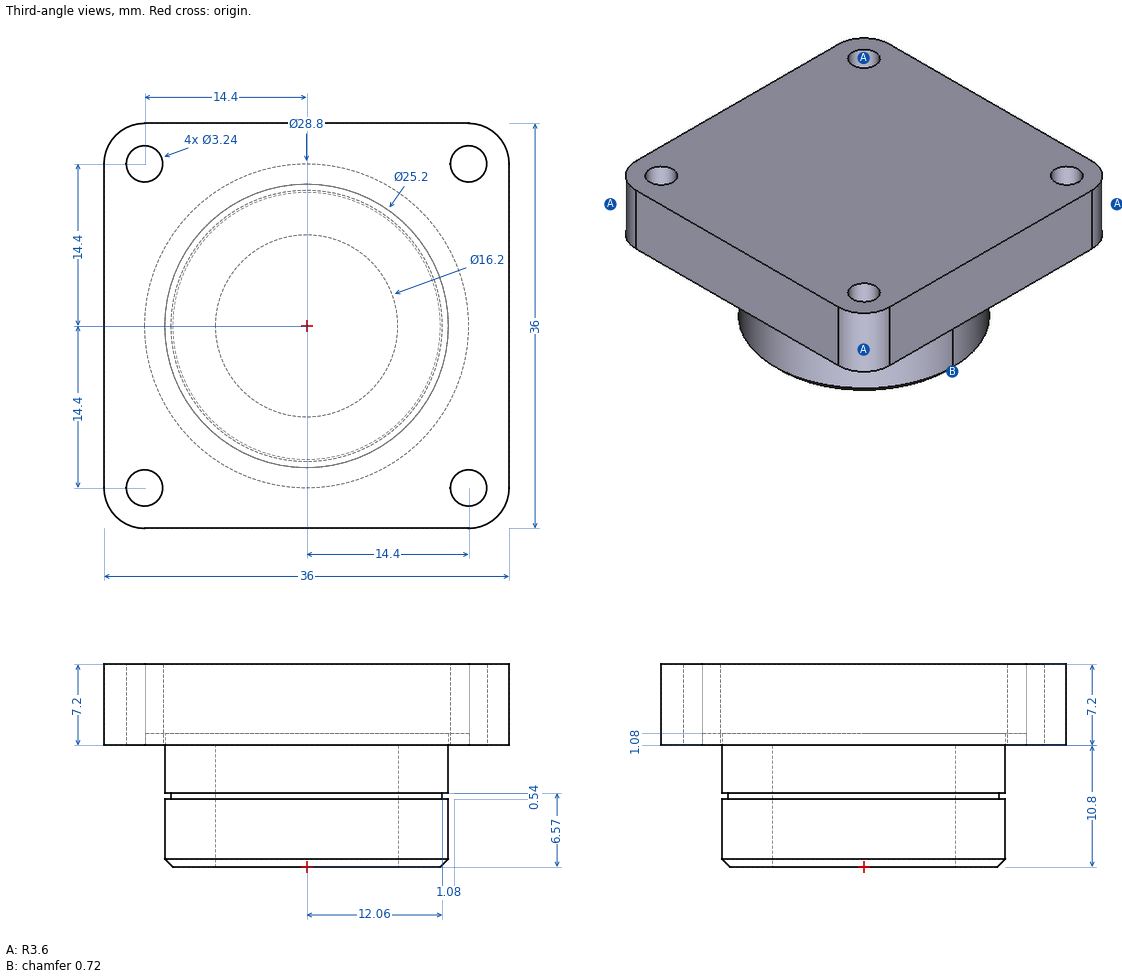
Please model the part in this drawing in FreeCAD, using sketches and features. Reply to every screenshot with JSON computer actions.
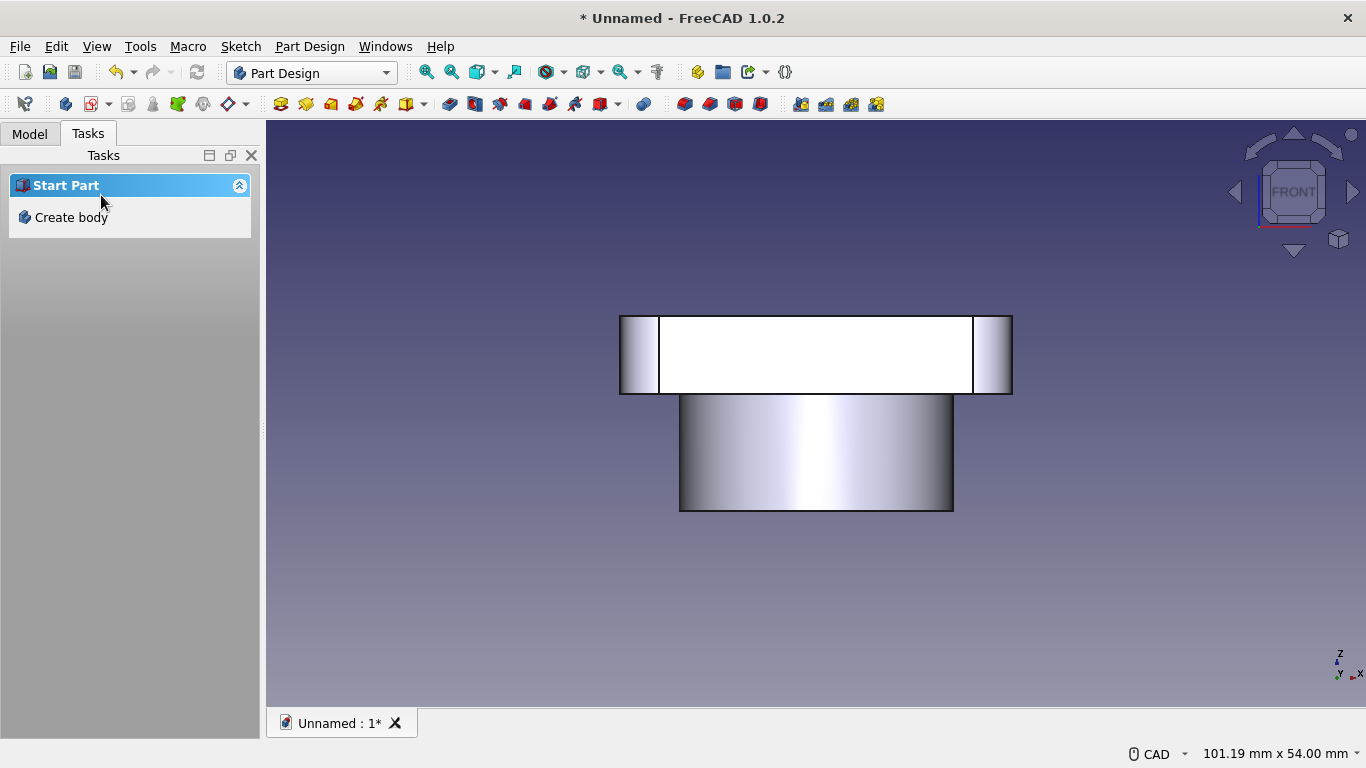
{"action": "left_click", "coordinate": [427, 72]}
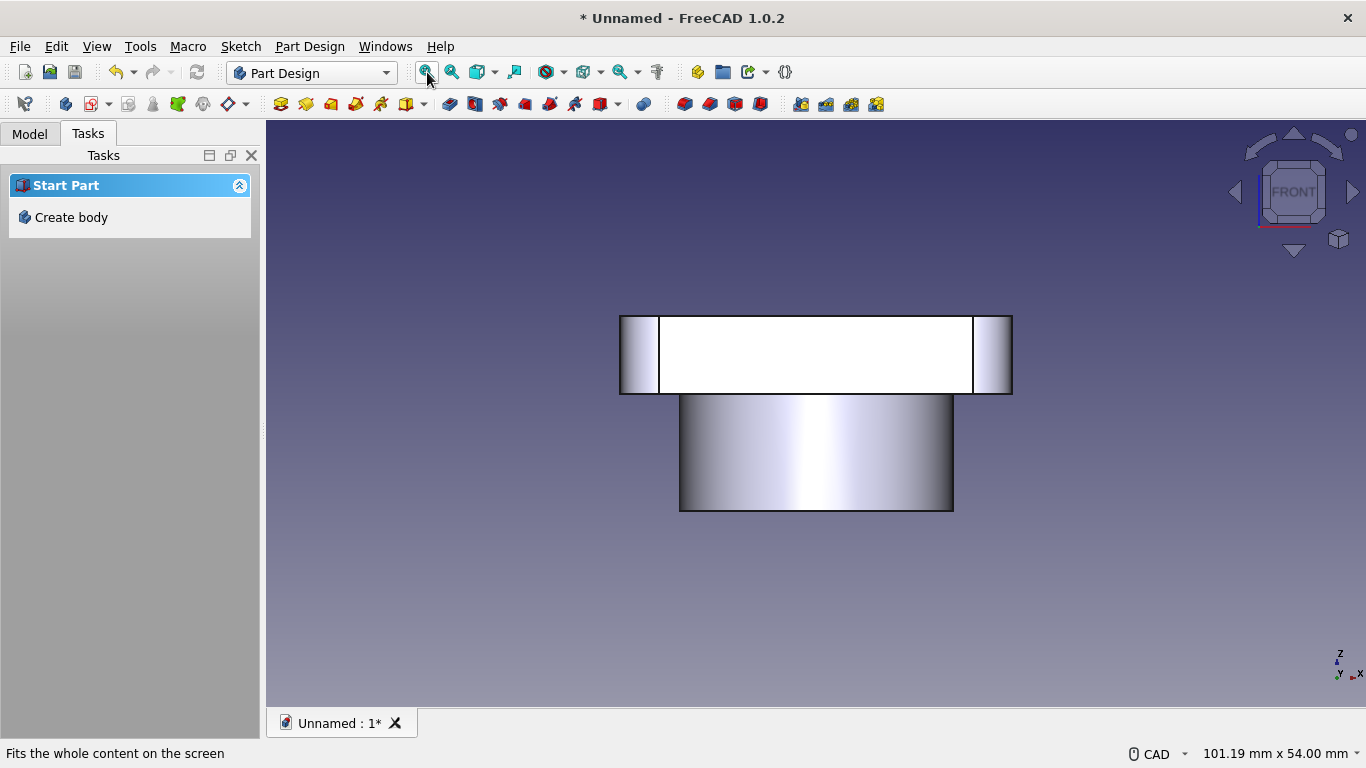
{"action": "key", "text": "3"}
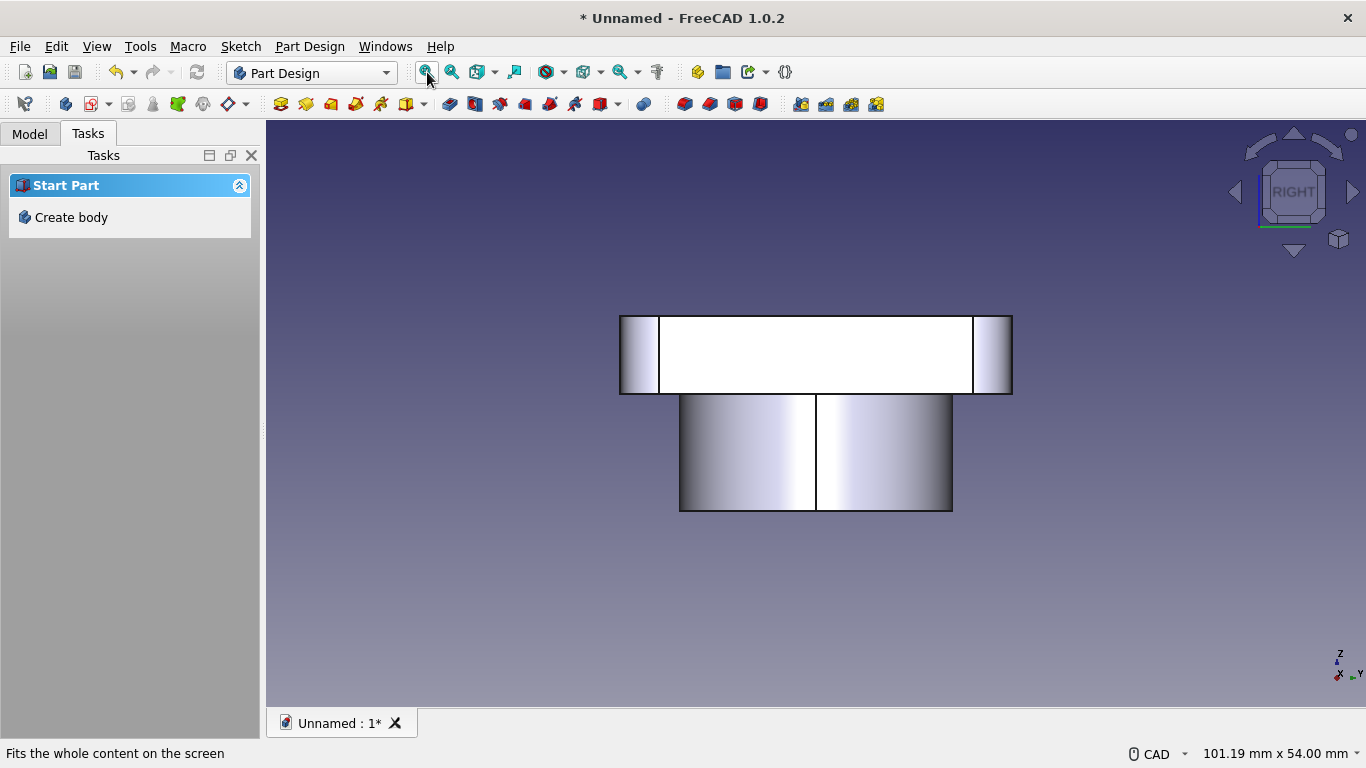
{"action": "left_click", "coordinate": [427, 72]}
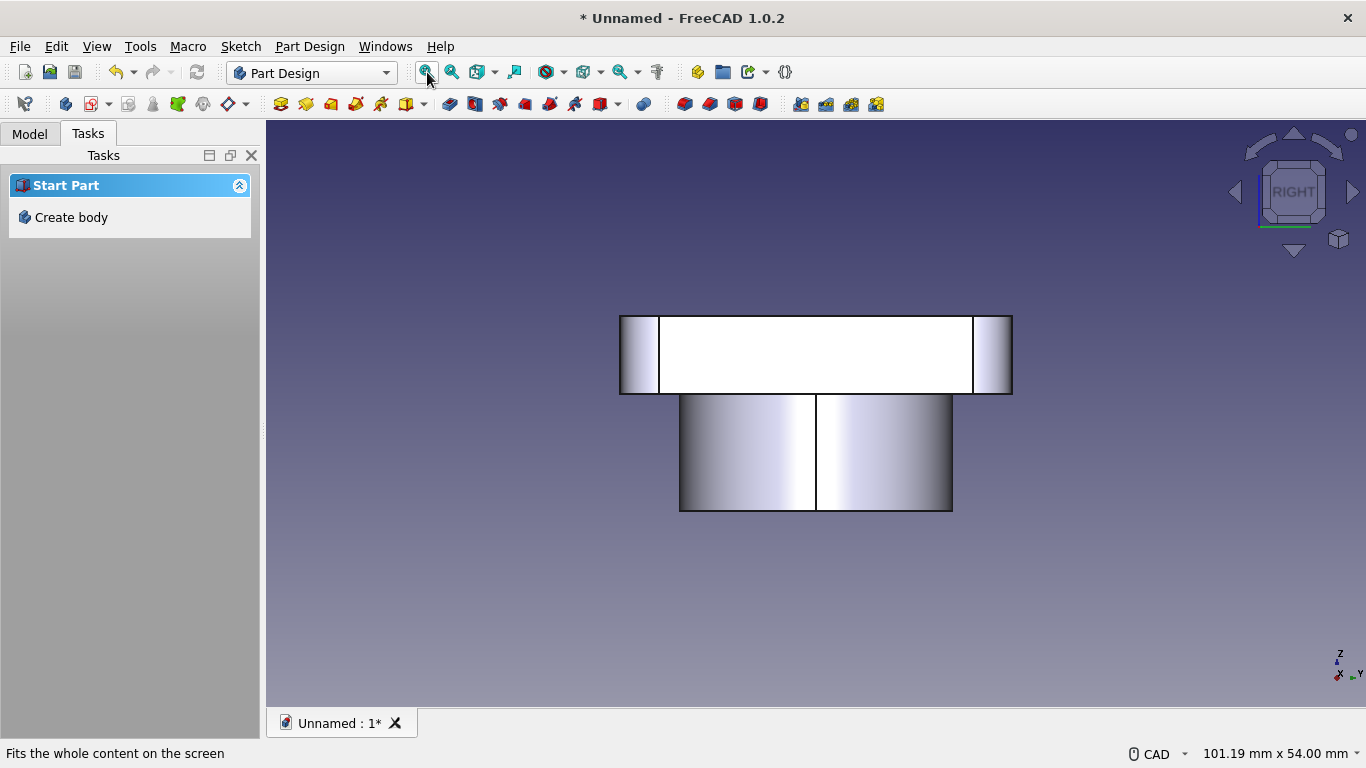
{"action": "key", "text": "5"}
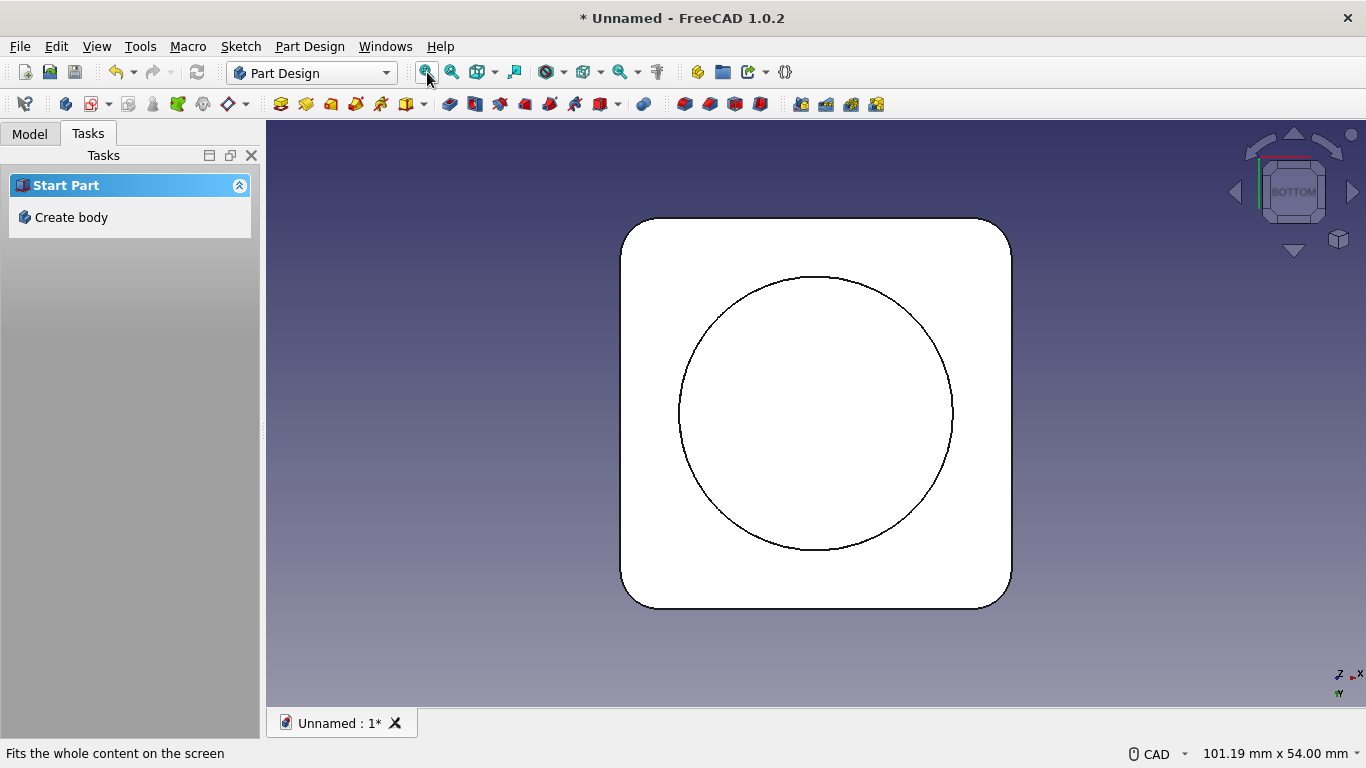
{"action": "left_click", "coordinate": [679, 412]}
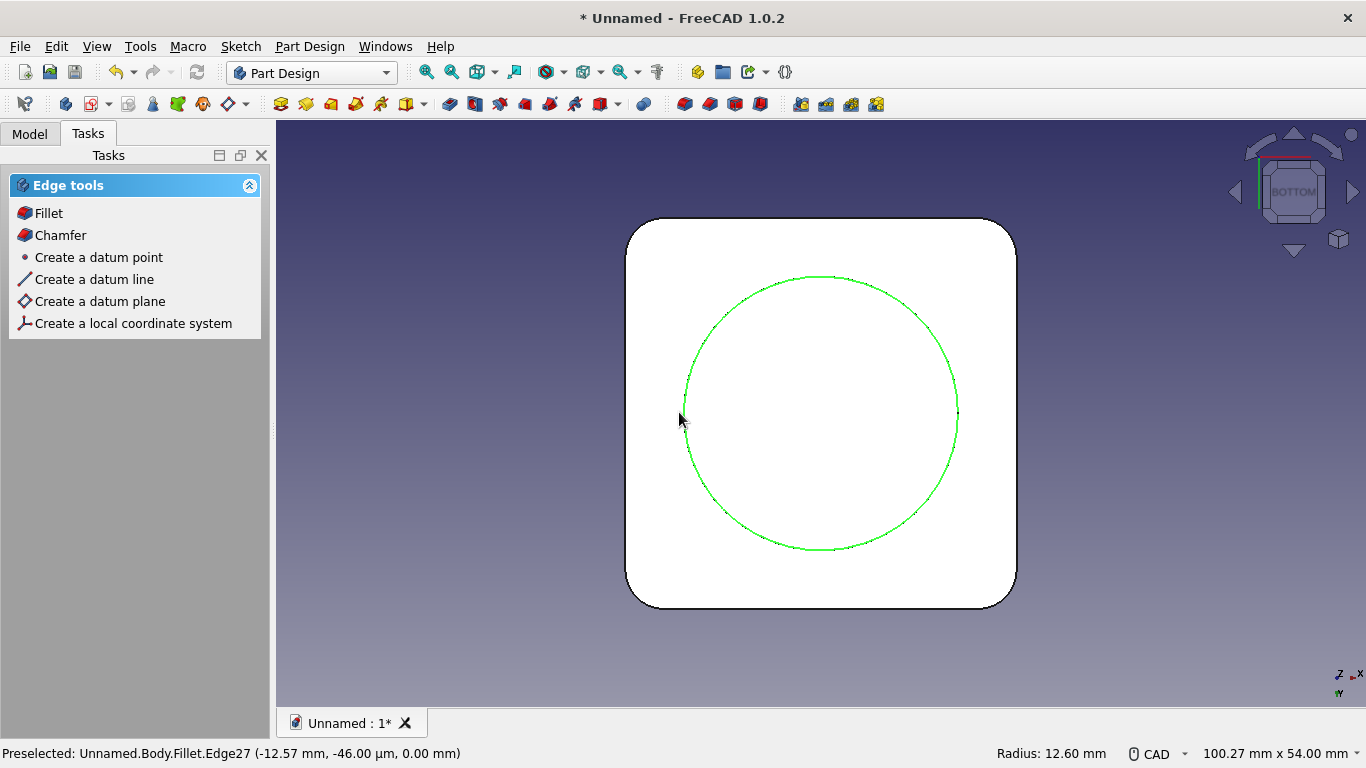
{"action": "left_click", "coordinate": [710, 104]}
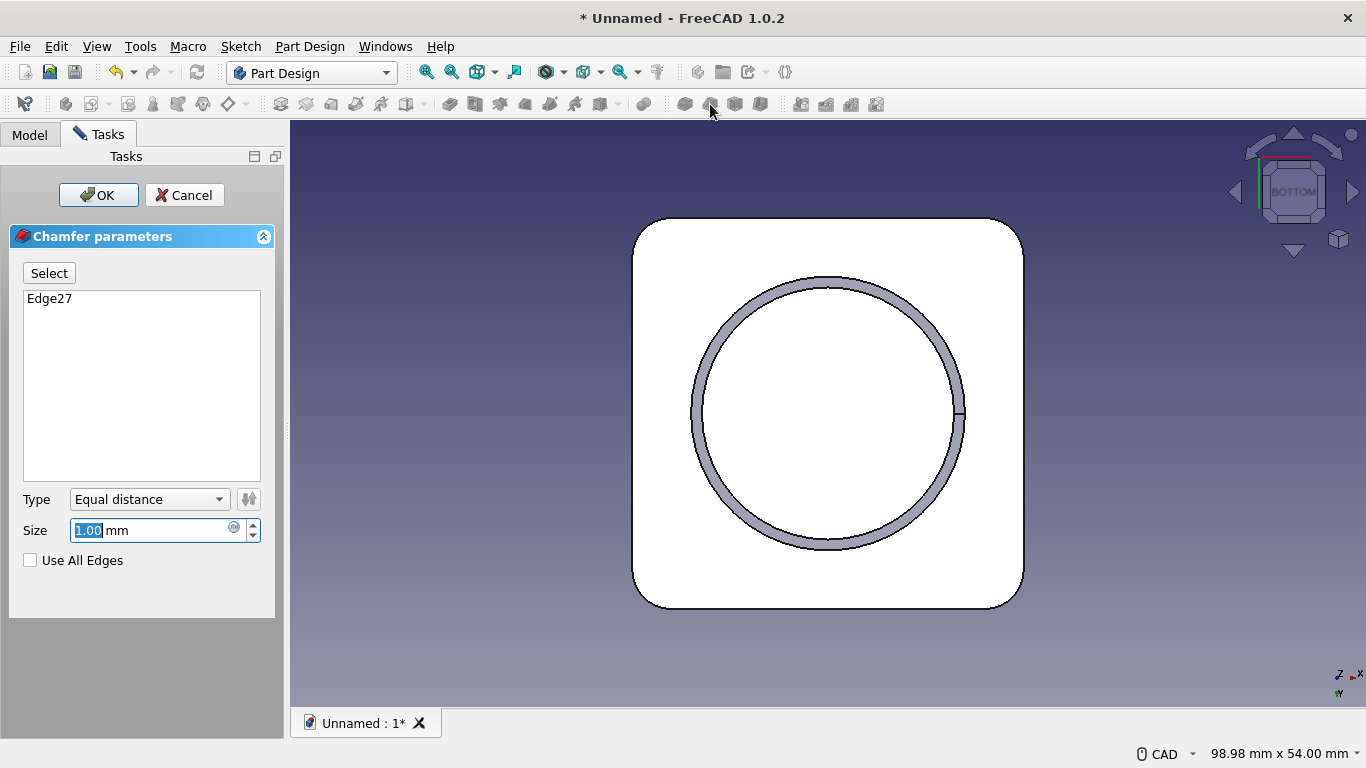
{"action": "type", "text": "0.72"}
{"action": "key", "text": "Tab"}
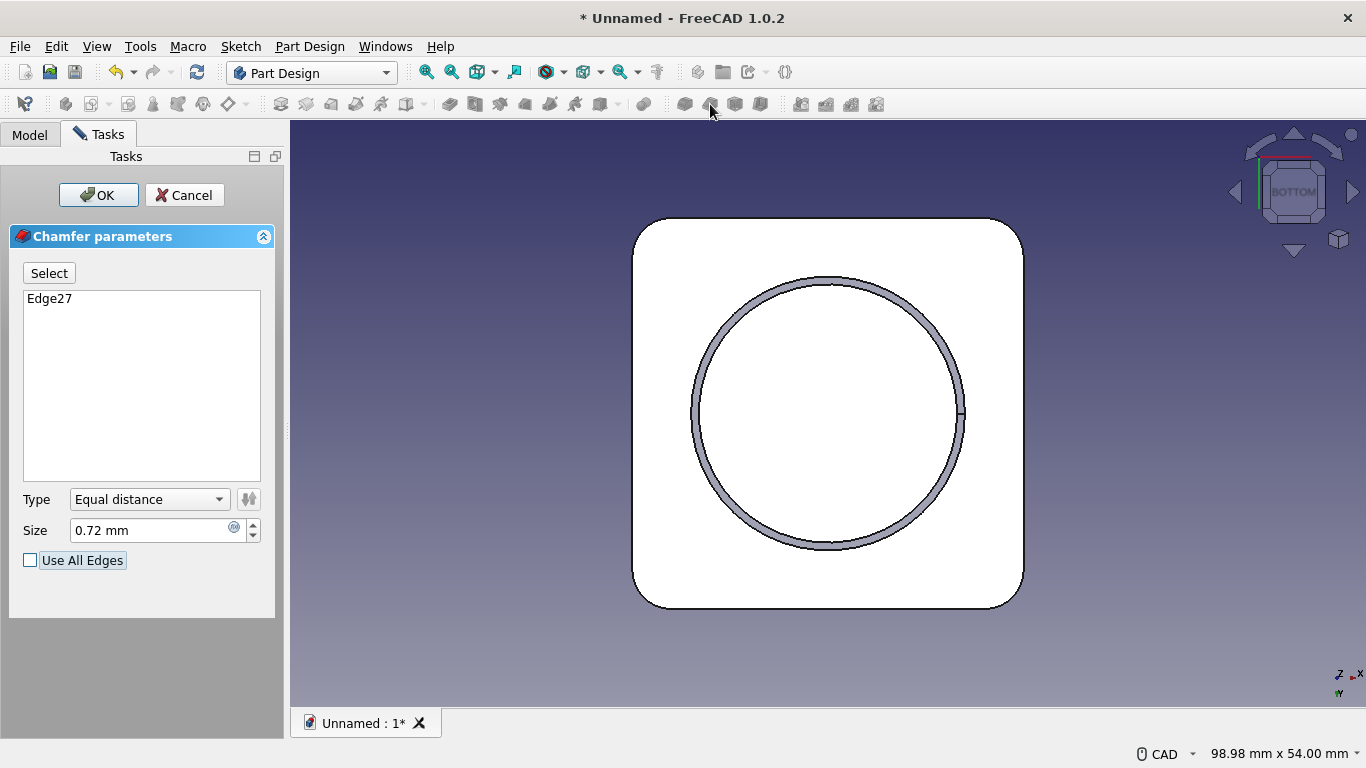
{"action": "left_click", "coordinate": [99, 195]}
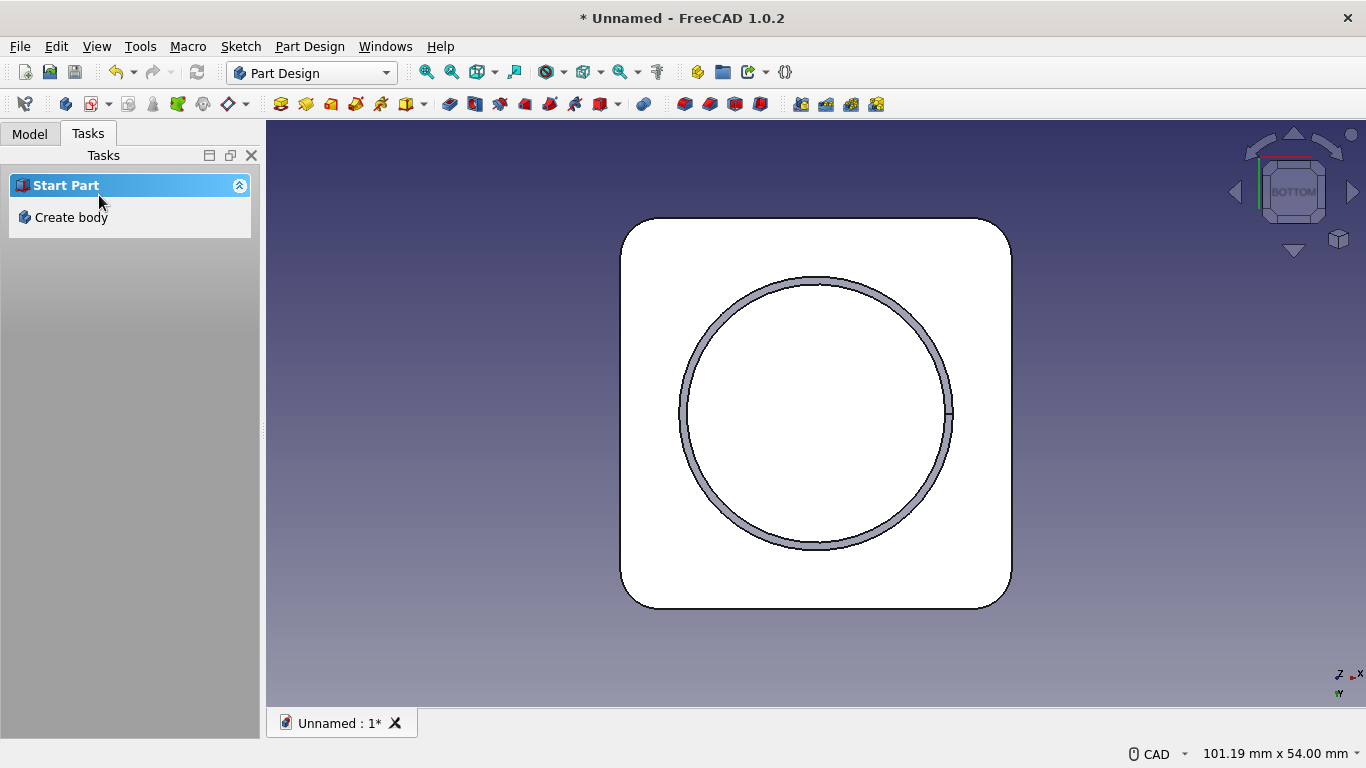
{"action": "left_click", "coordinate": [928, 245]}